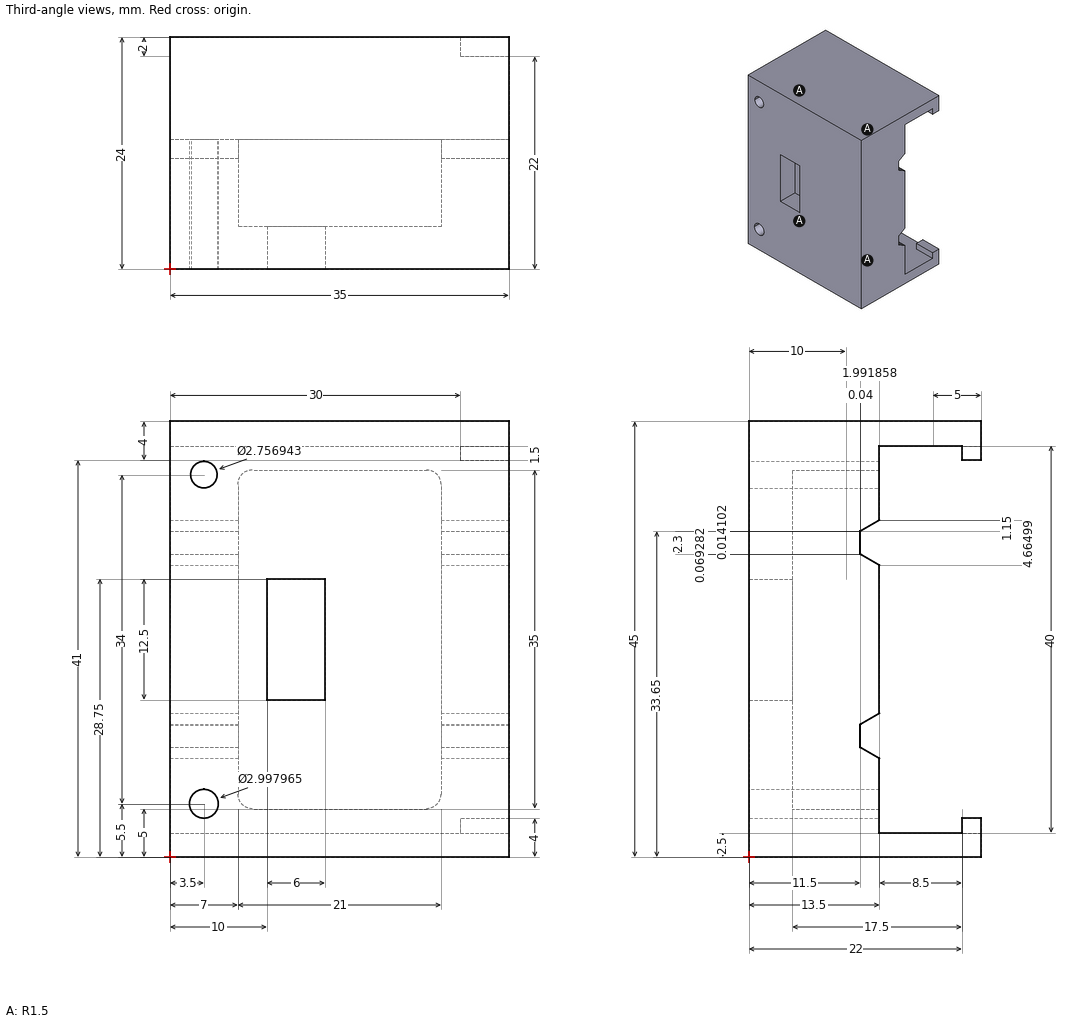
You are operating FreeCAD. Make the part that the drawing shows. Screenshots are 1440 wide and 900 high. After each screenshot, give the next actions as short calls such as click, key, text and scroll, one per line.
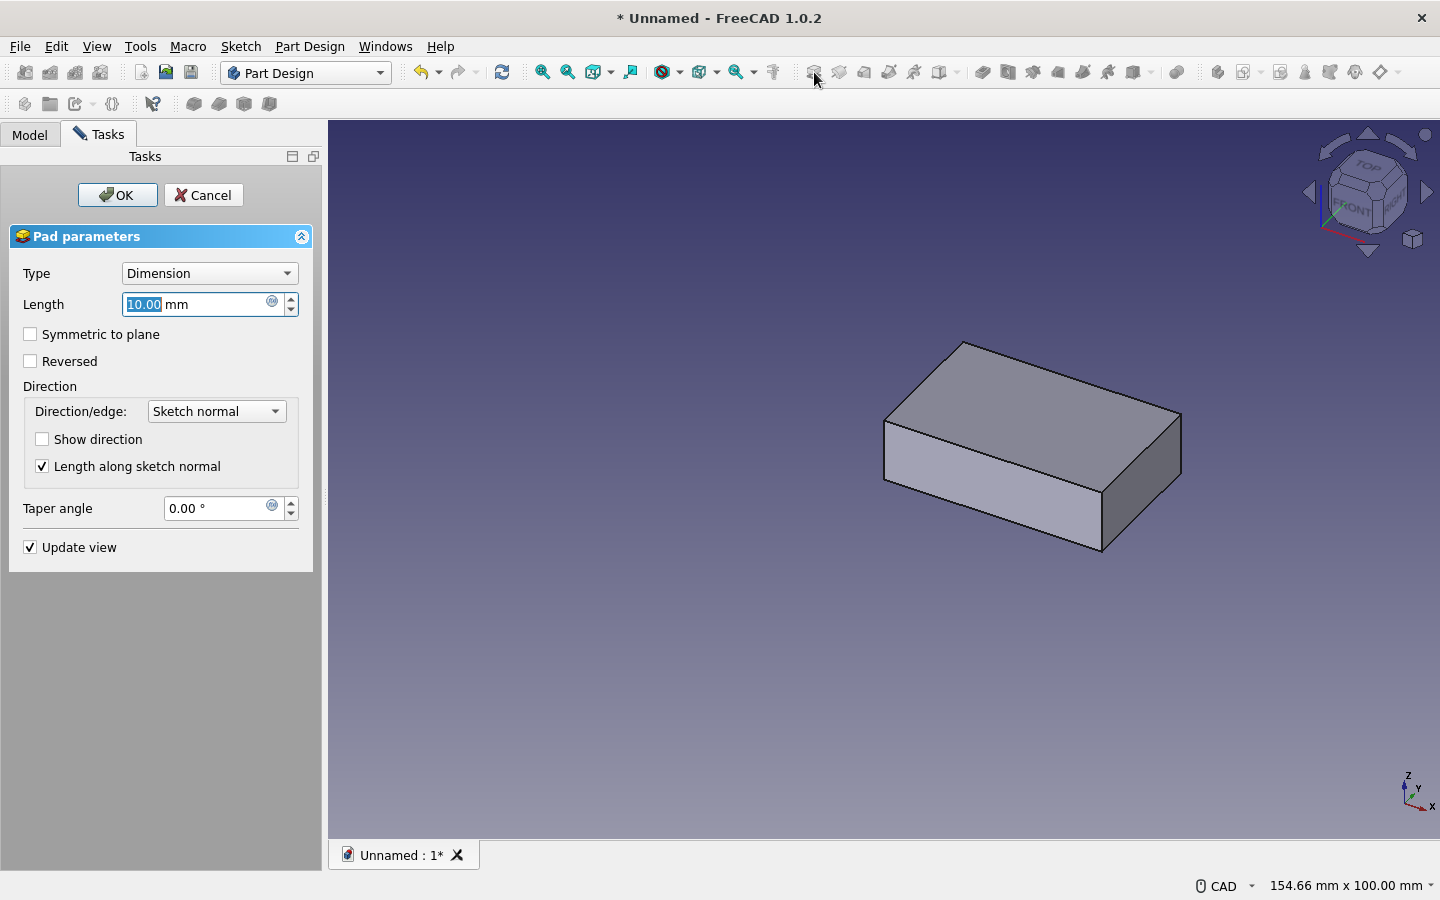
text(45)
key(Tab)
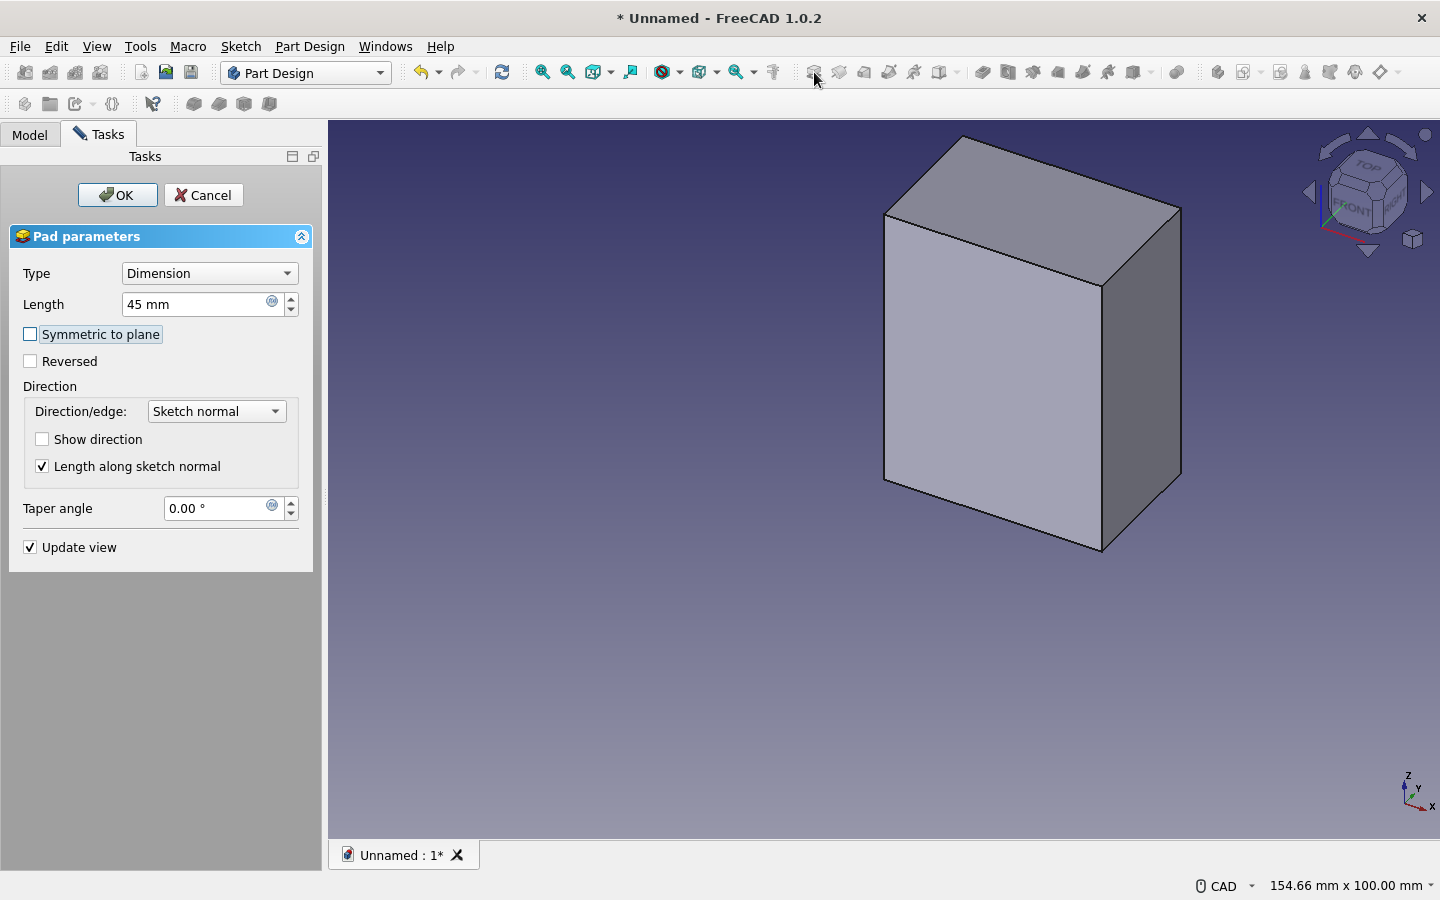
click(118, 195)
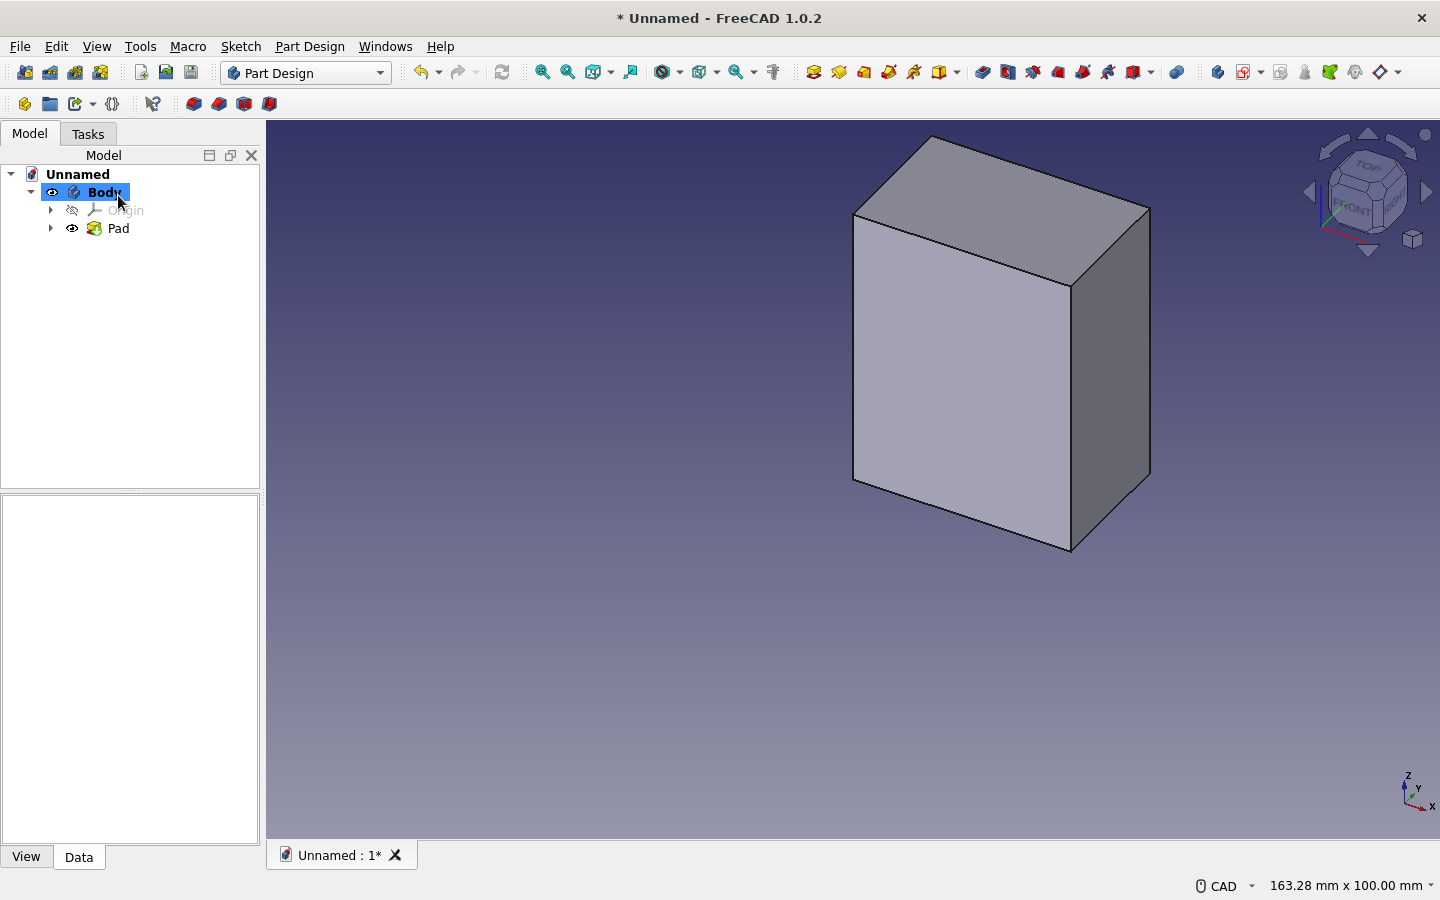
key(4)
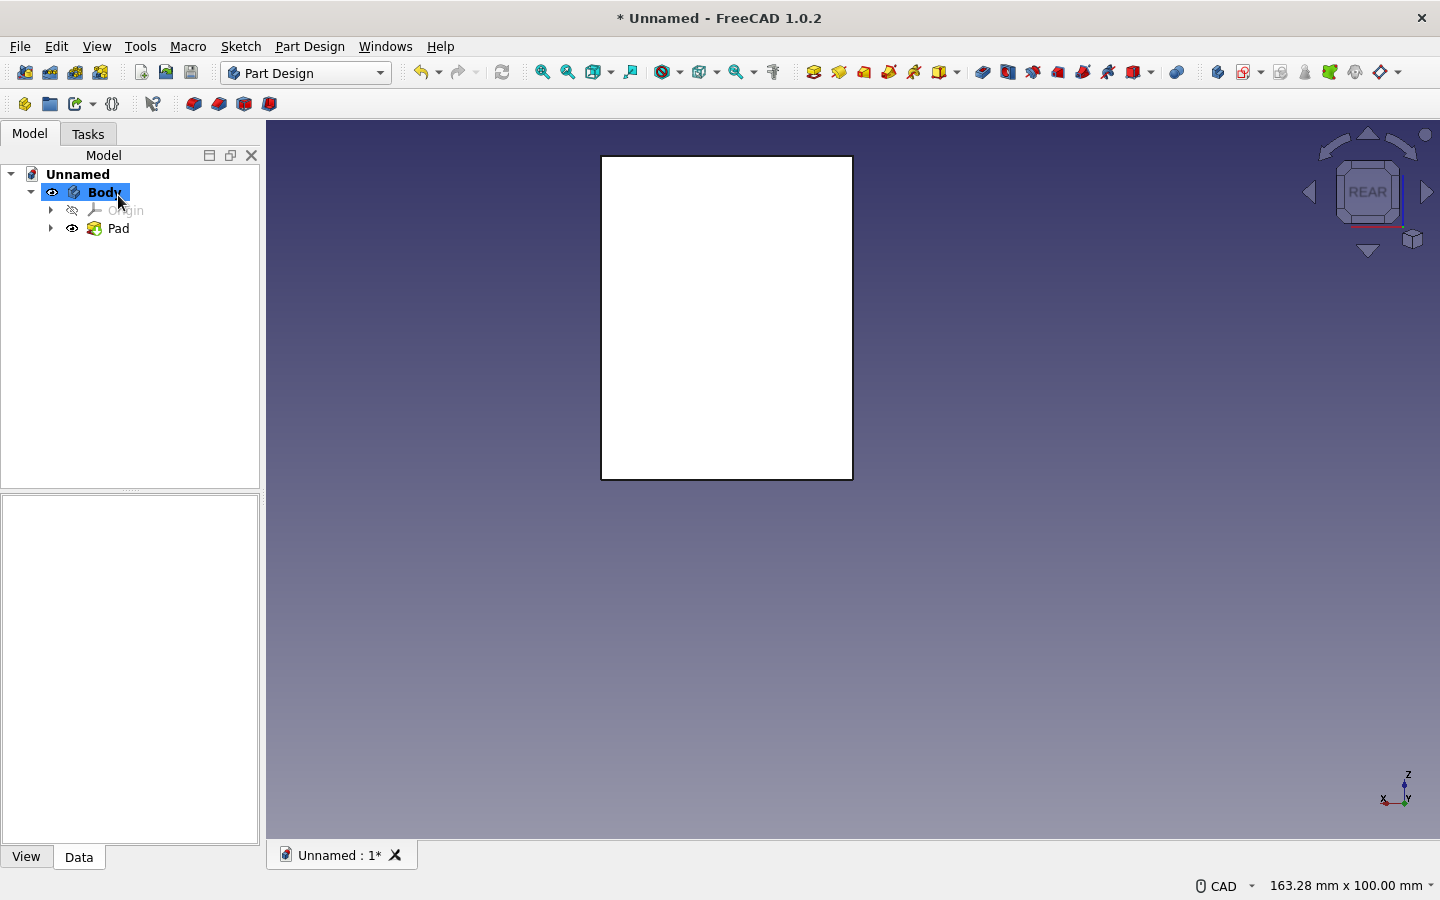
click(543, 72)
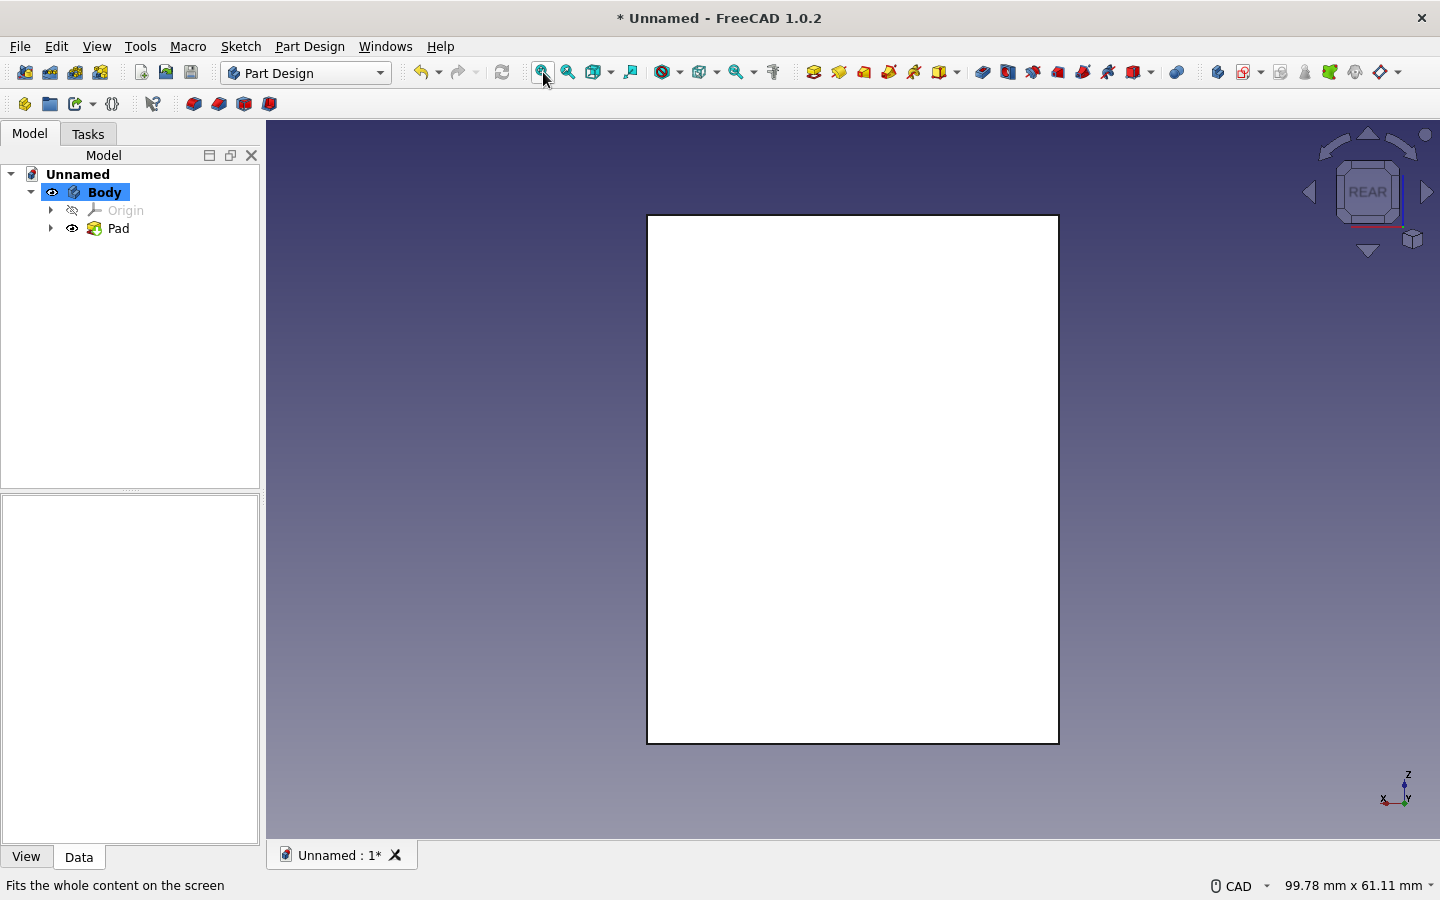
click(853, 479)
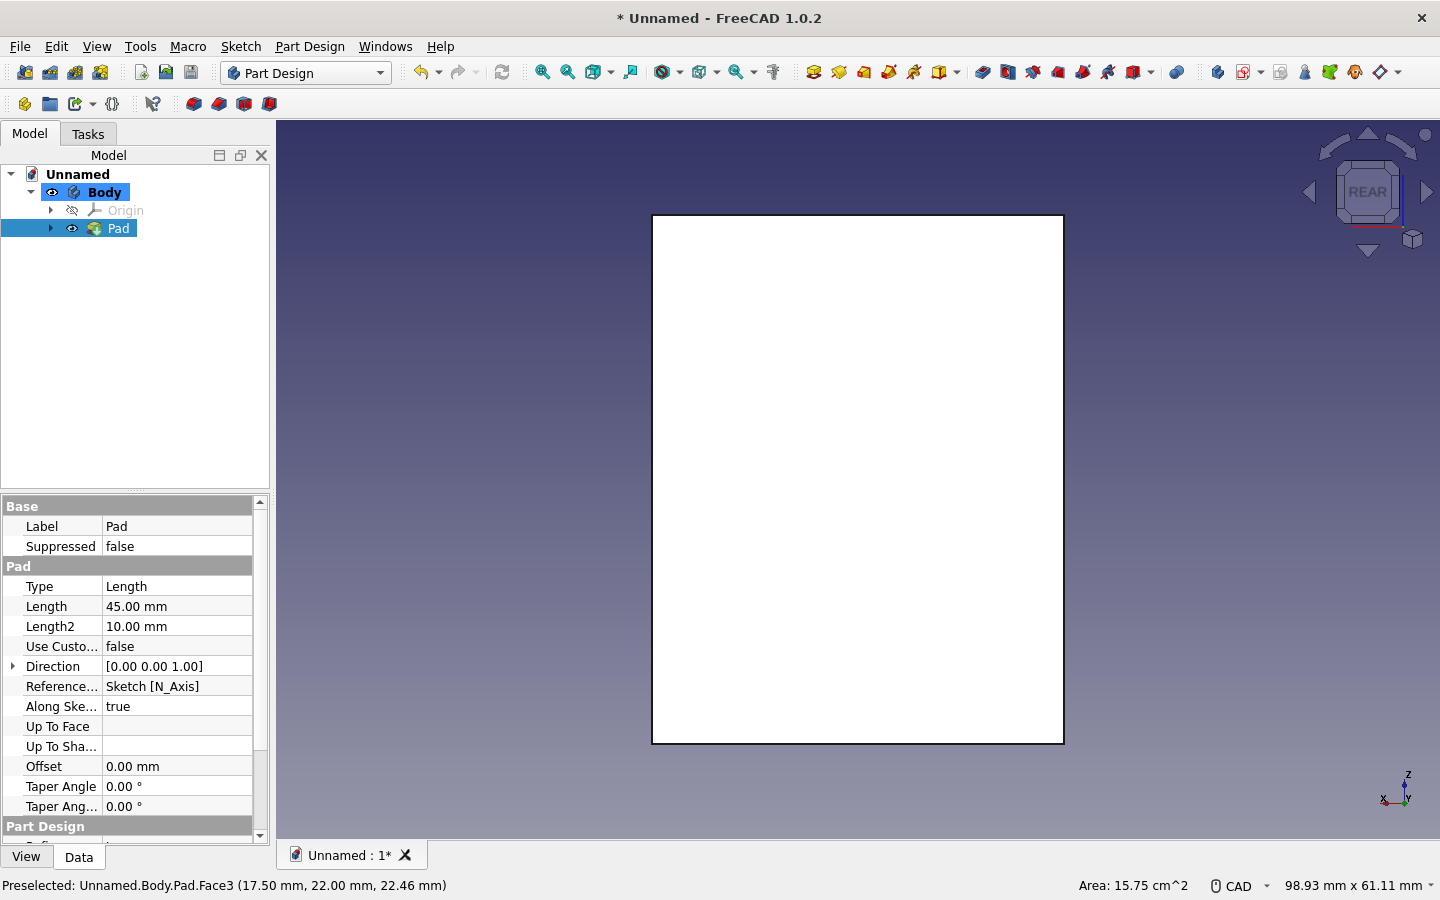
click(1242, 72)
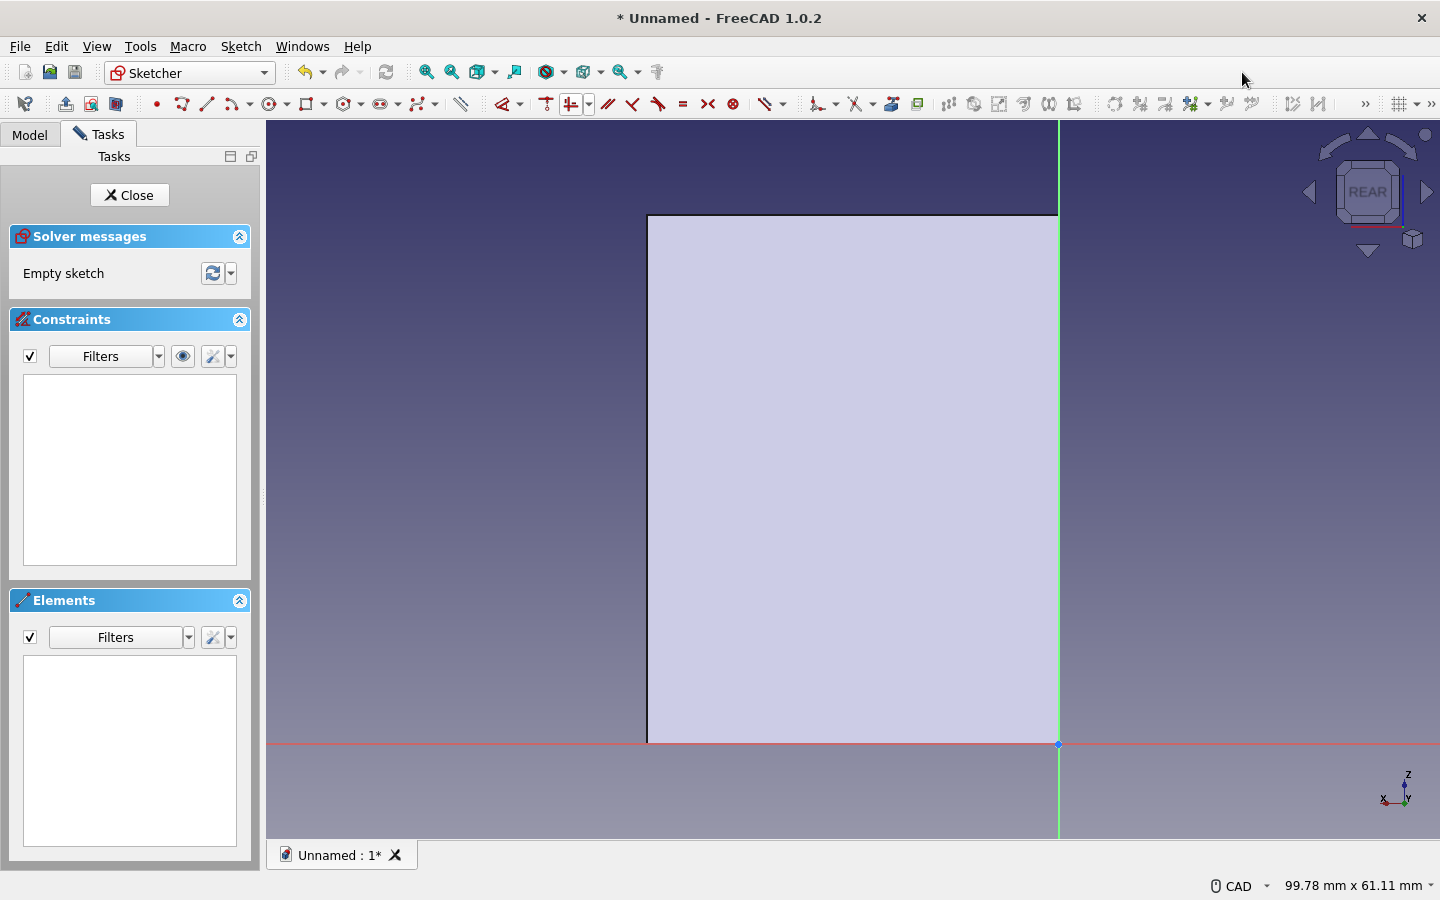
click(306, 104)